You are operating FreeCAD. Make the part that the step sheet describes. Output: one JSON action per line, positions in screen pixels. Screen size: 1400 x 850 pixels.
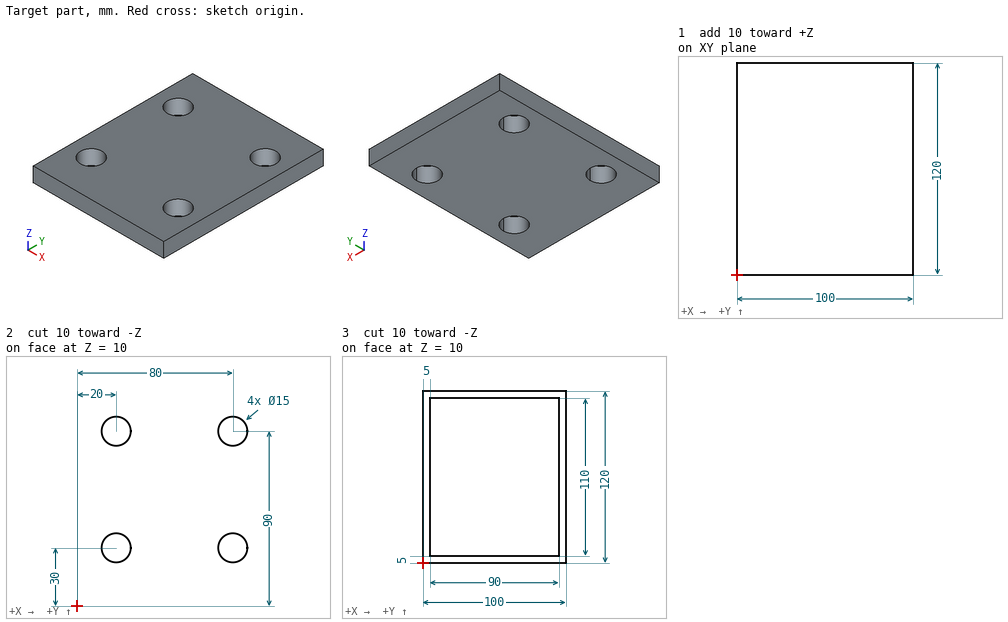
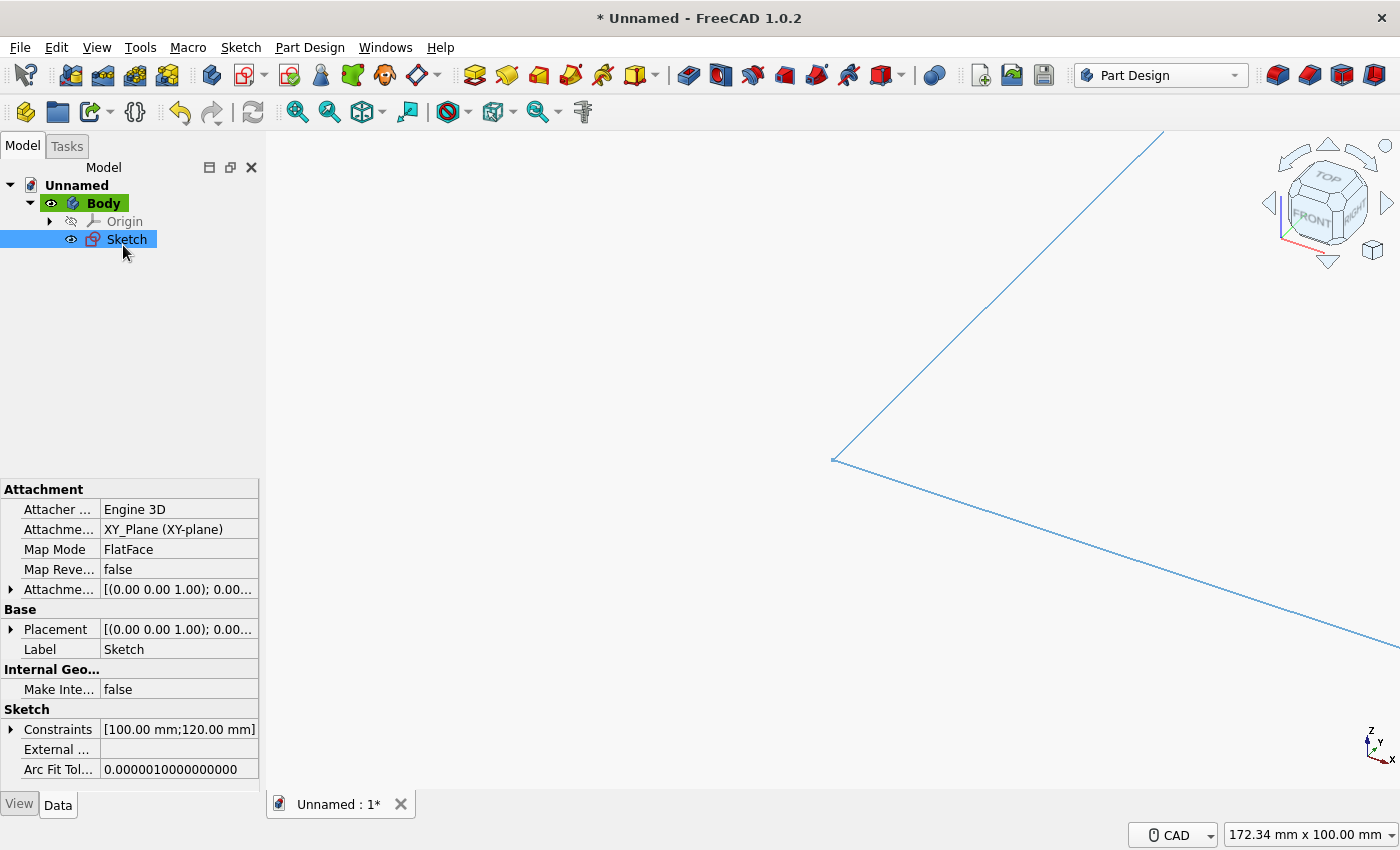
{"action": "left_click", "coordinate": [476, 76]}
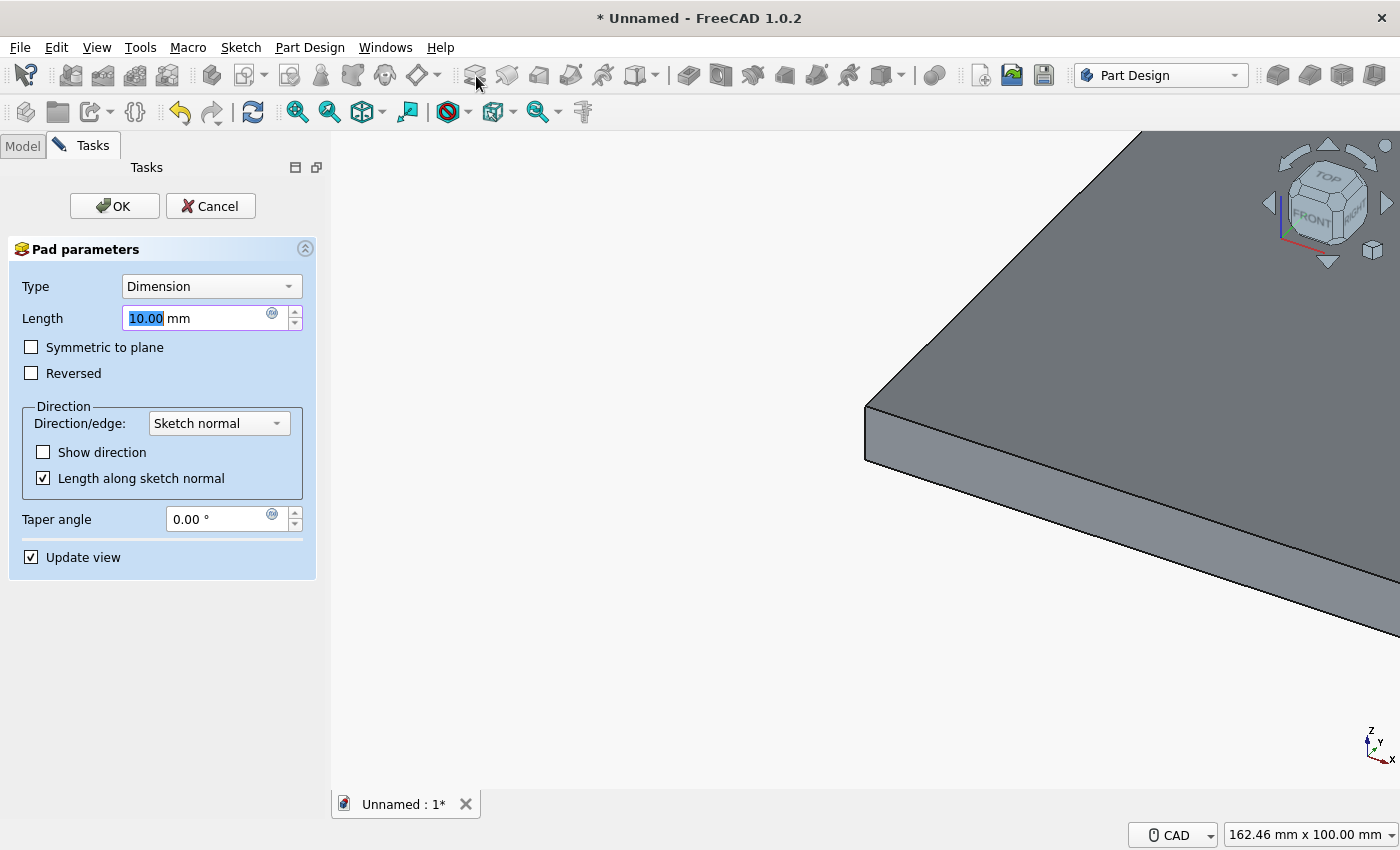
{"action": "type", "text": "10"}
{"action": "key", "text": "Tab"}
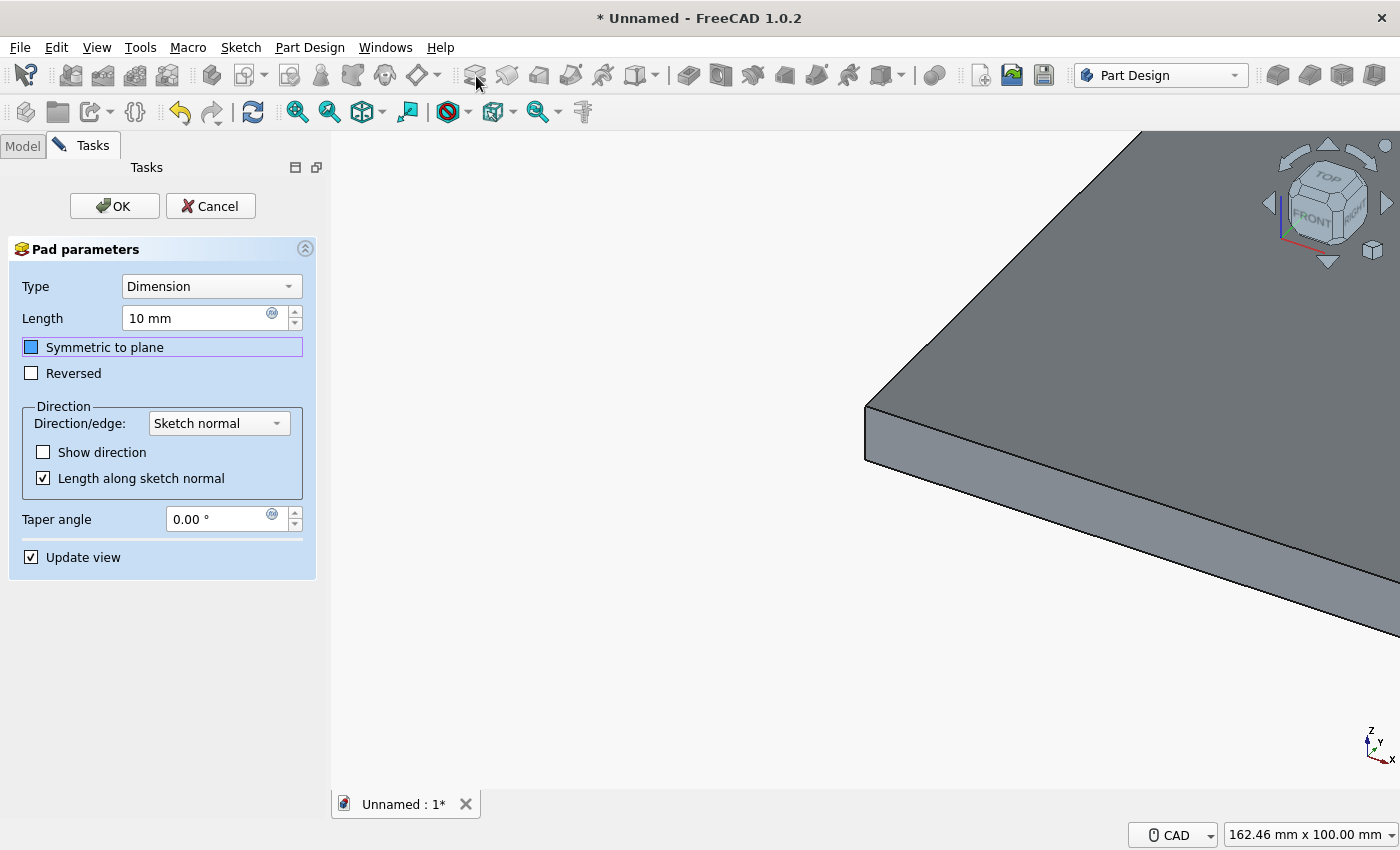
{"action": "left_click", "coordinate": [115, 206]}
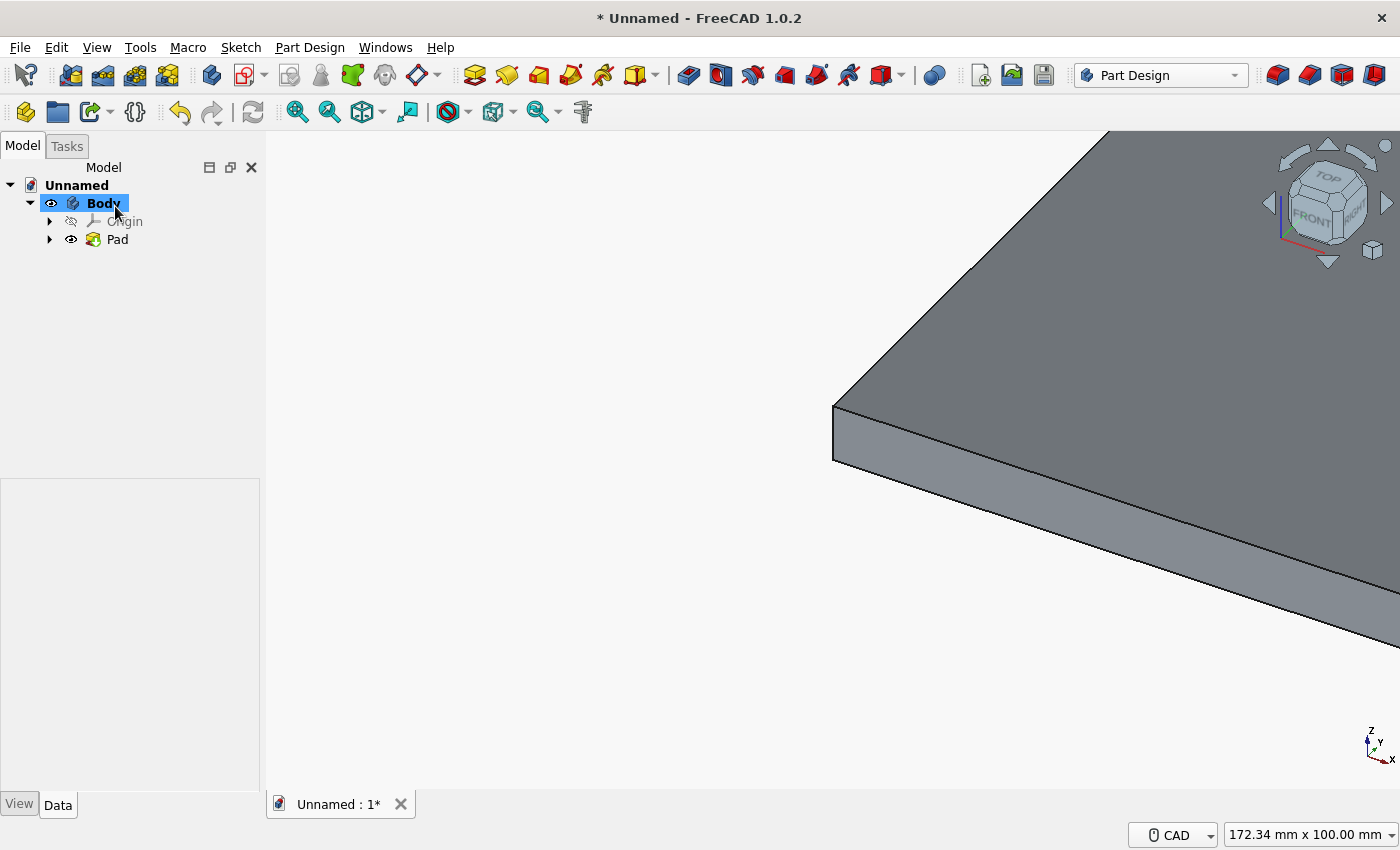
{"action": "key", "text": "v f"}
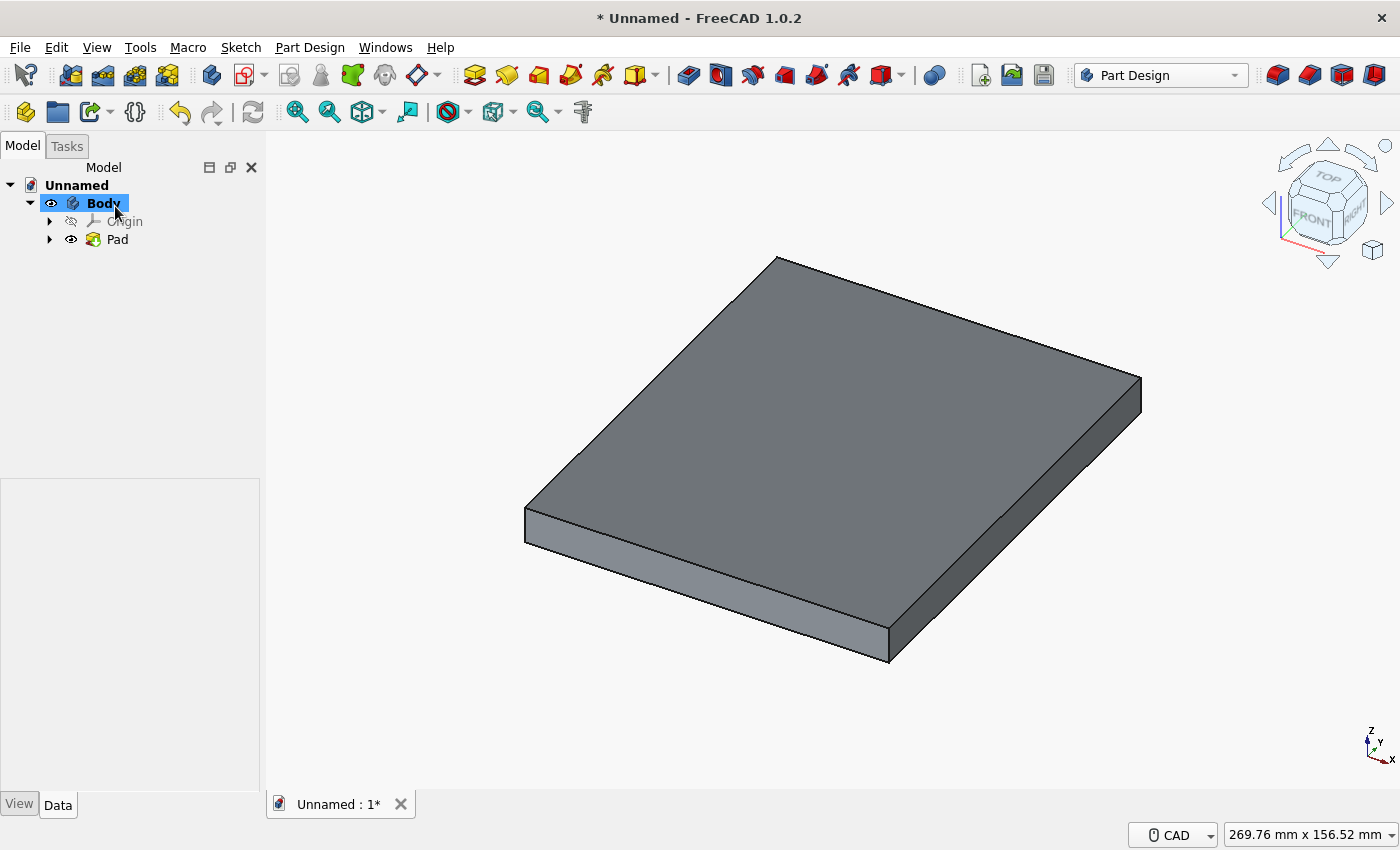
{"action": "left_click", "coordinate": [833, 442]}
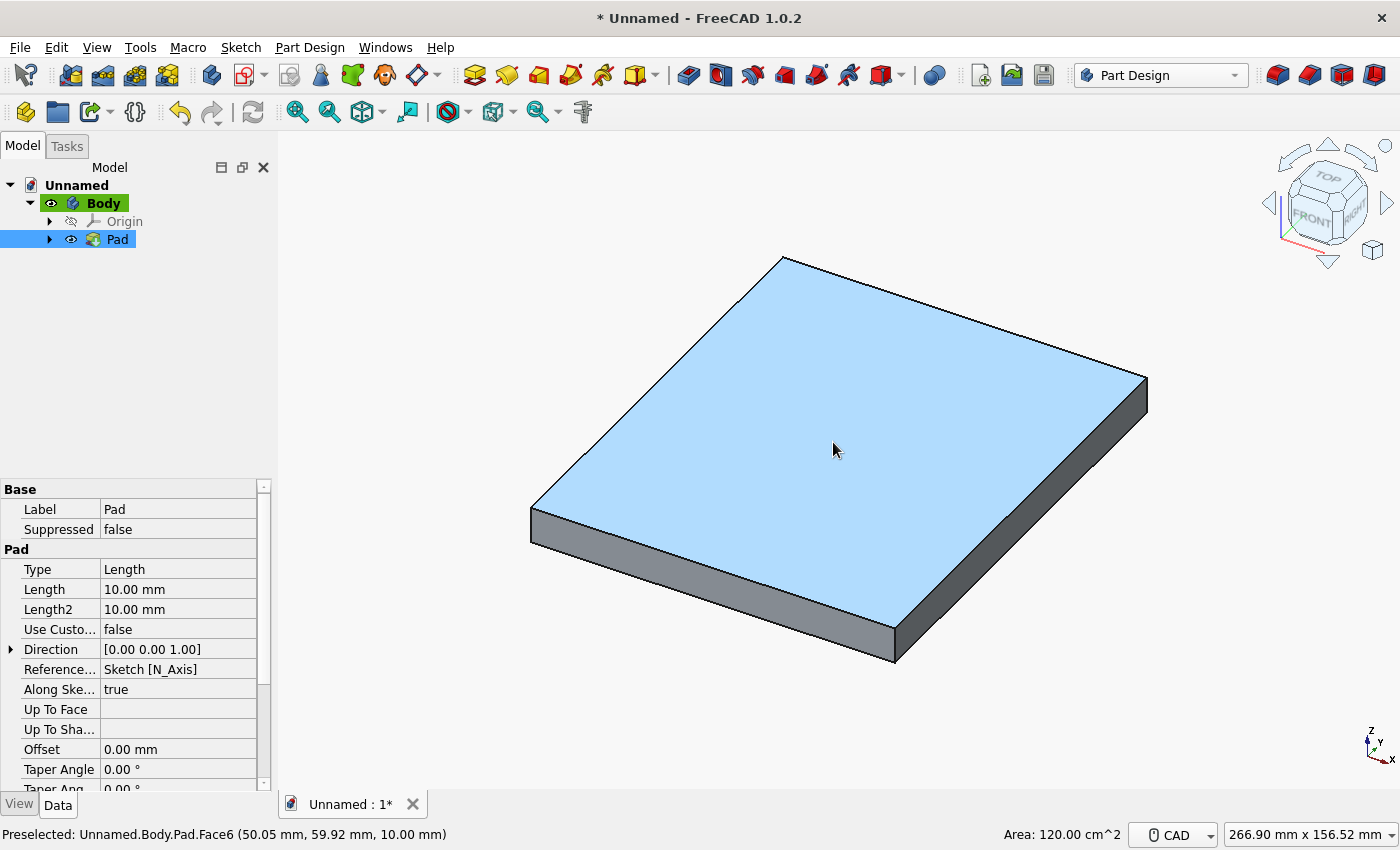
{"action": "left_click", "coordinate": [244, 76]}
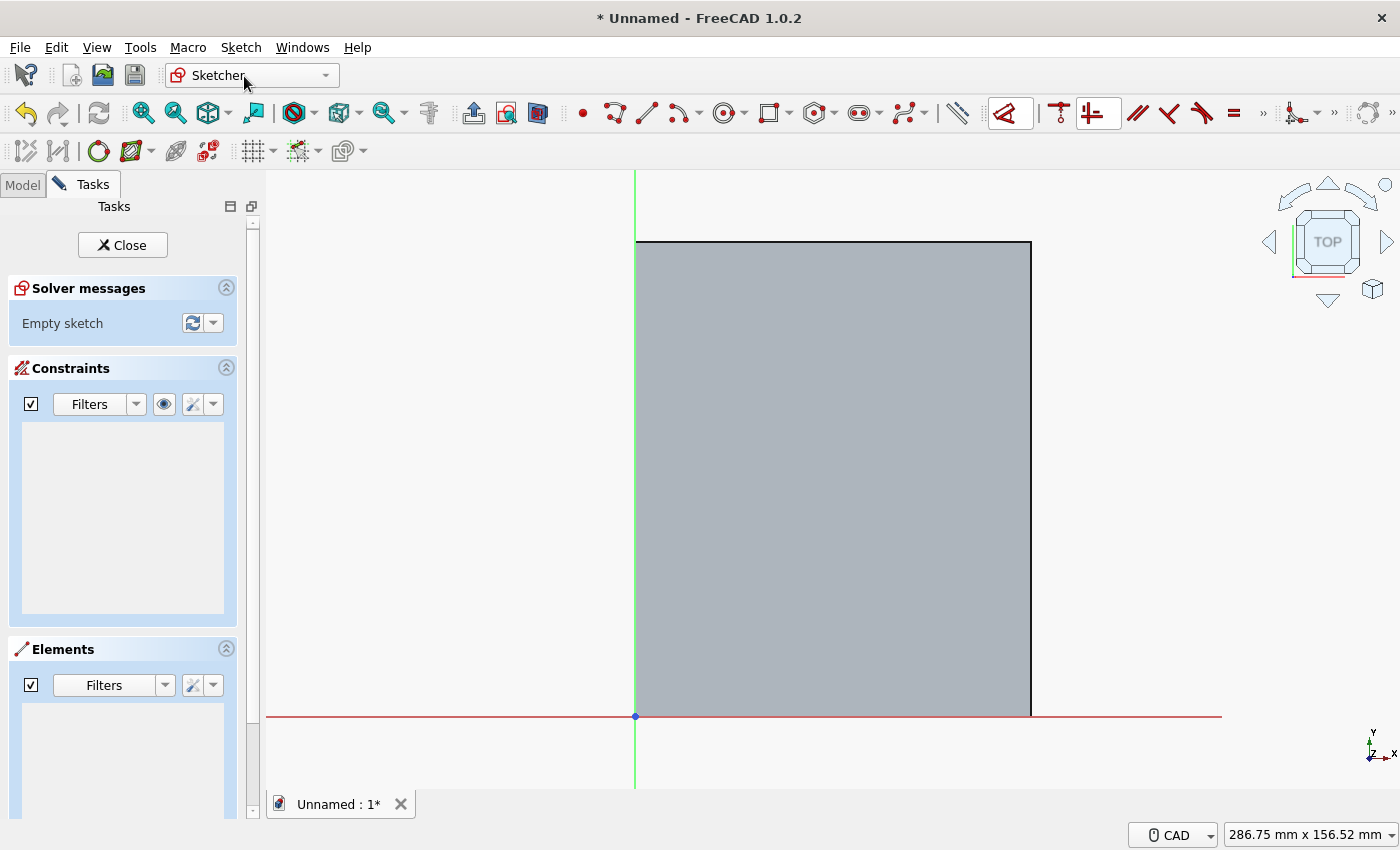
{"action": "key", "text": "g c"}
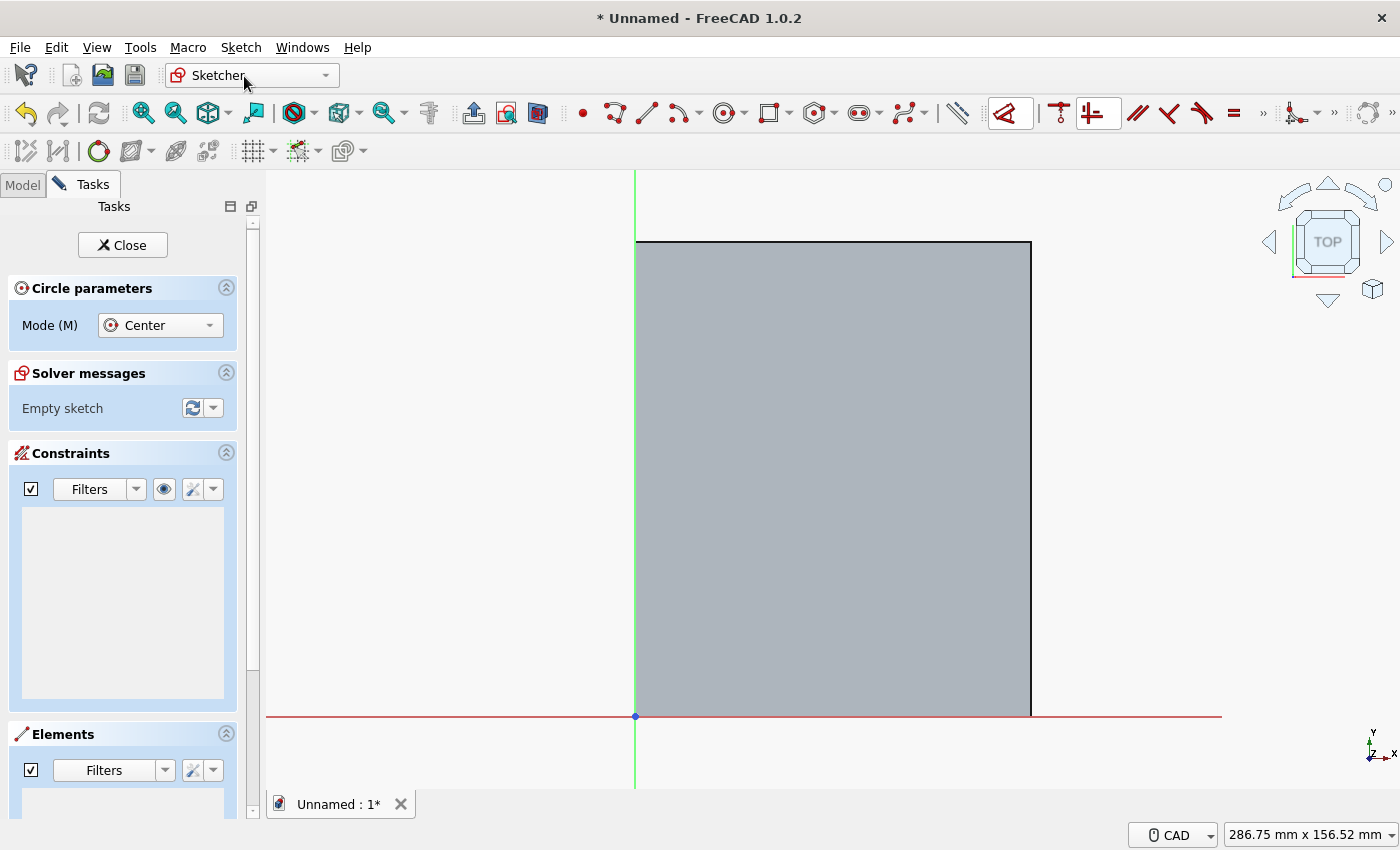
{"action": "left_click", "coordinate": [952, 361]}
{"action": "mouse_move", "coordinate": [973, 340]}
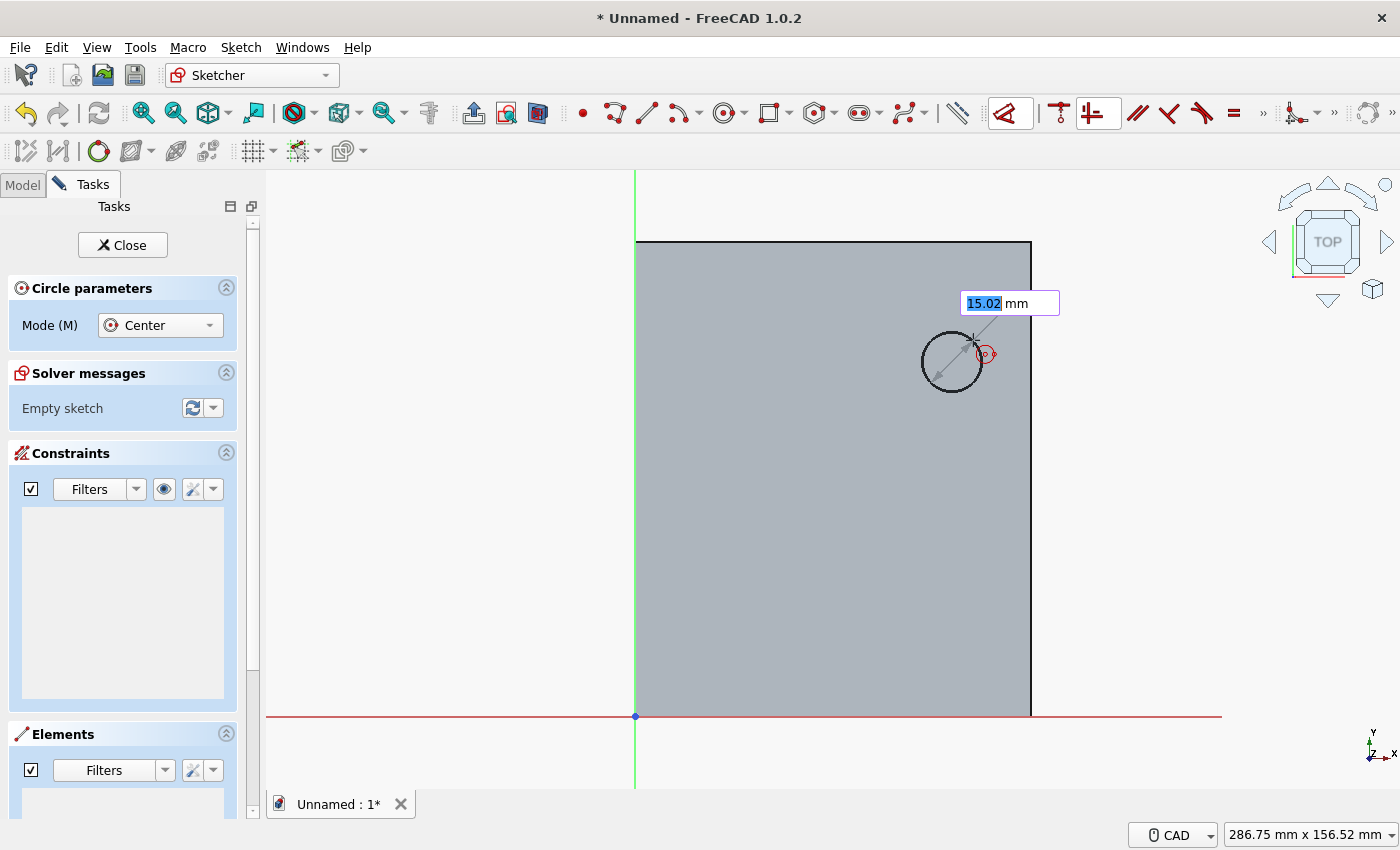
{"action": "type", "text": "15"}
{"action": "key", "text": "Return"}